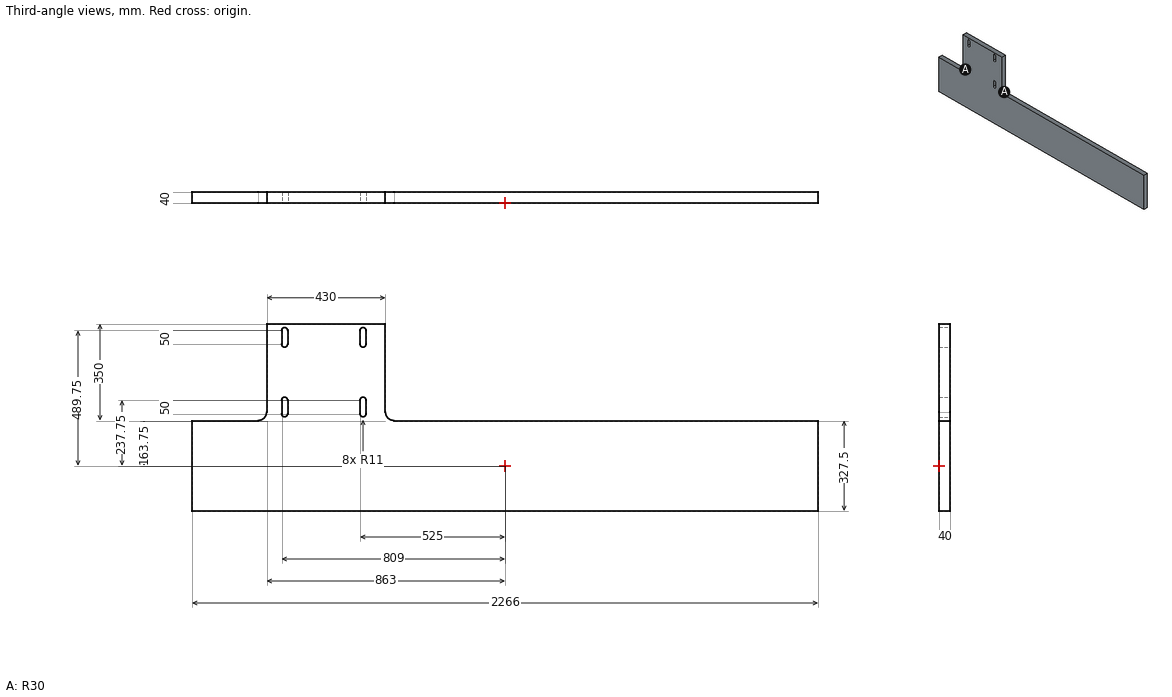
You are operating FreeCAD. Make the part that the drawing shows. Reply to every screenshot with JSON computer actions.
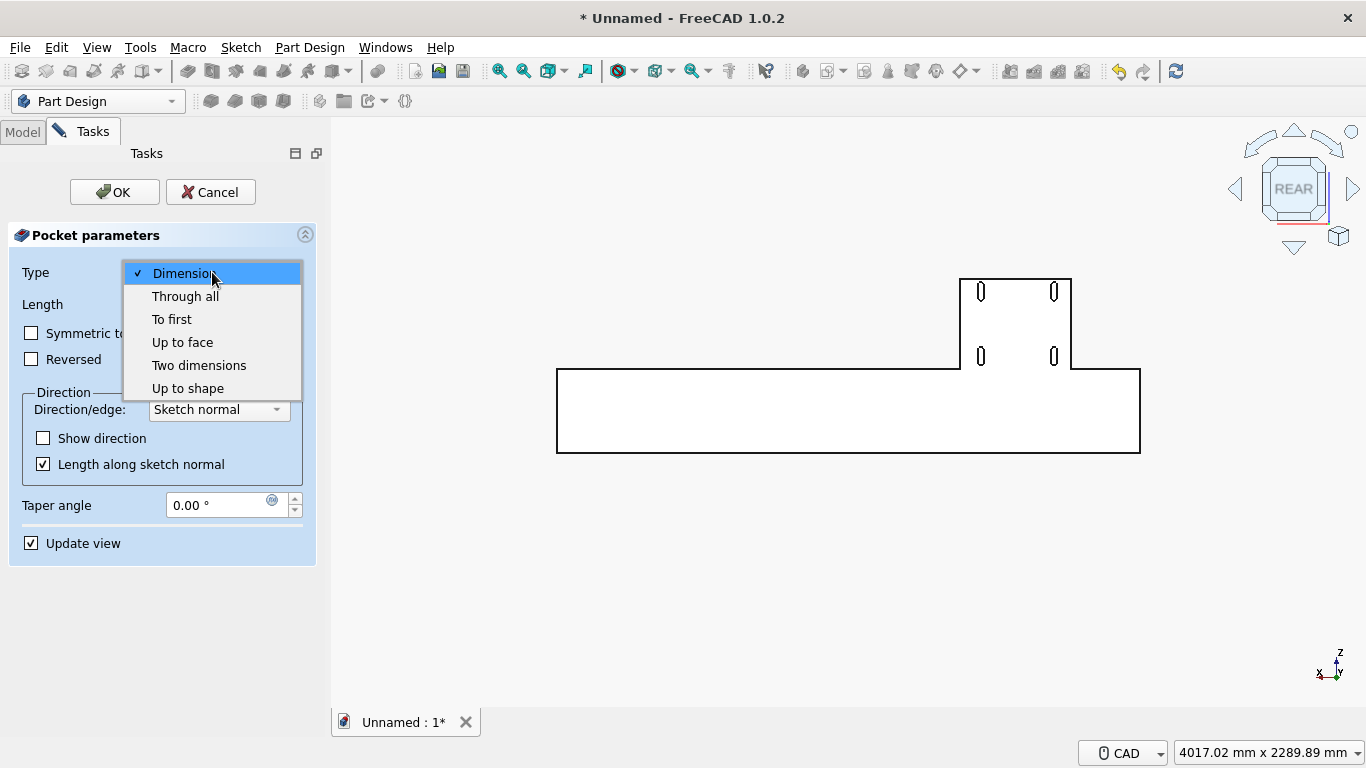
{"action": "left_click", "coordinate": [212, 296]}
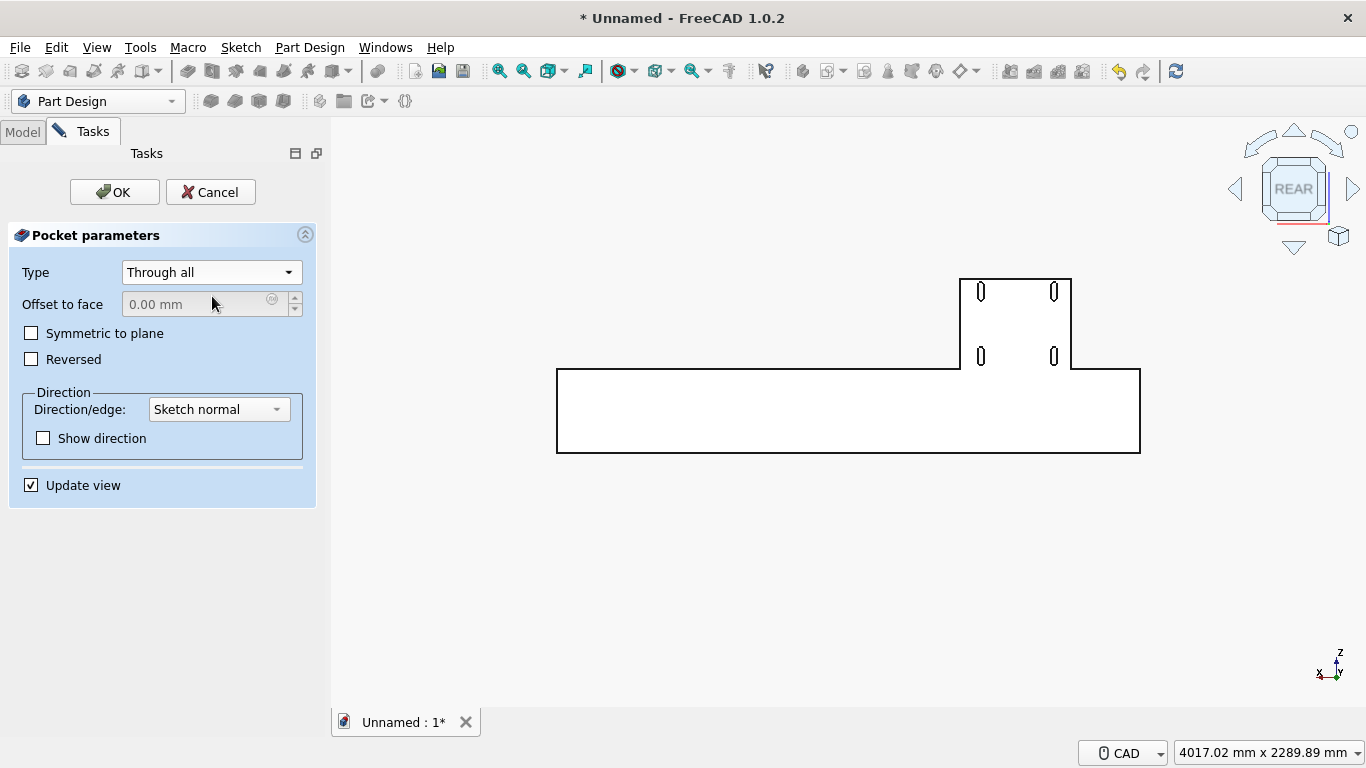
{"action": "left_click", "coordinate": [115, 192]}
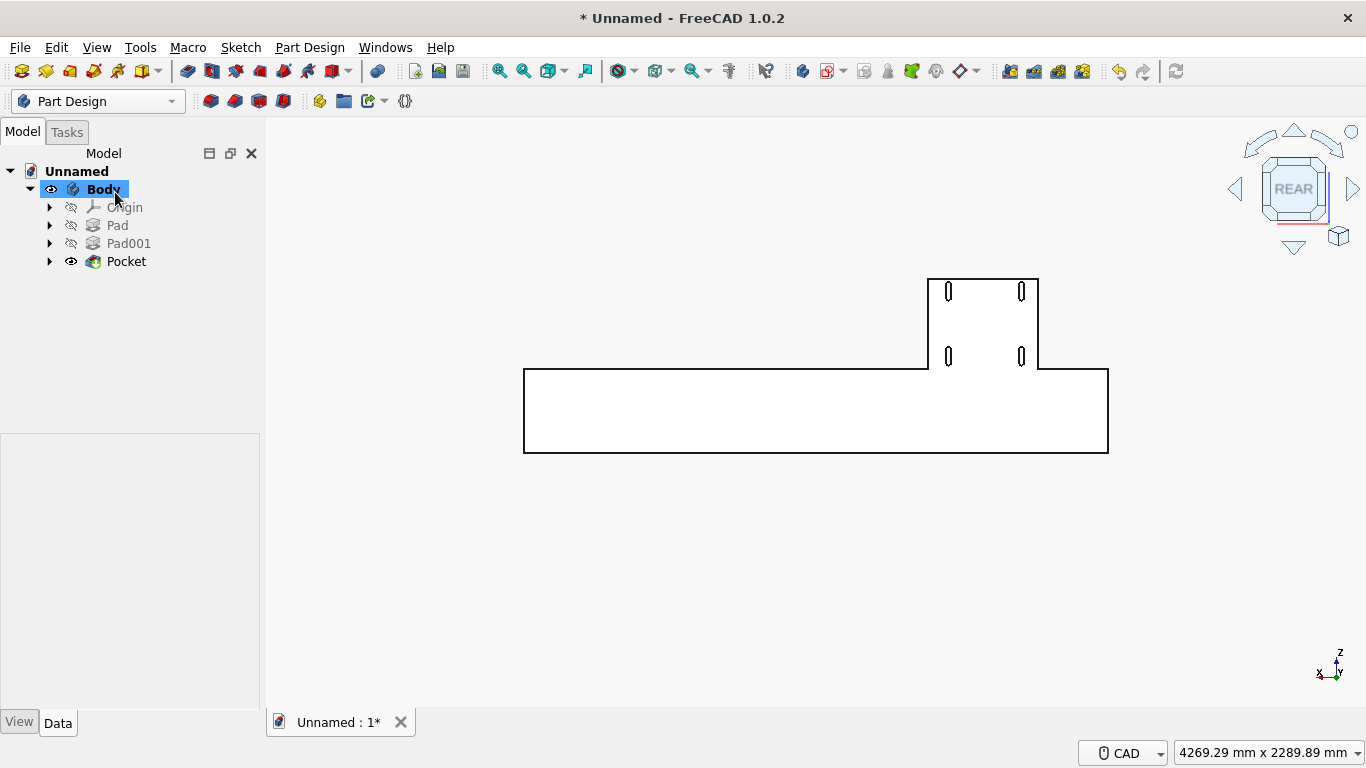
{"action": "scroll", "coordinate": [928, 368], "scroll_direction": "up", "scroll_amount": 7}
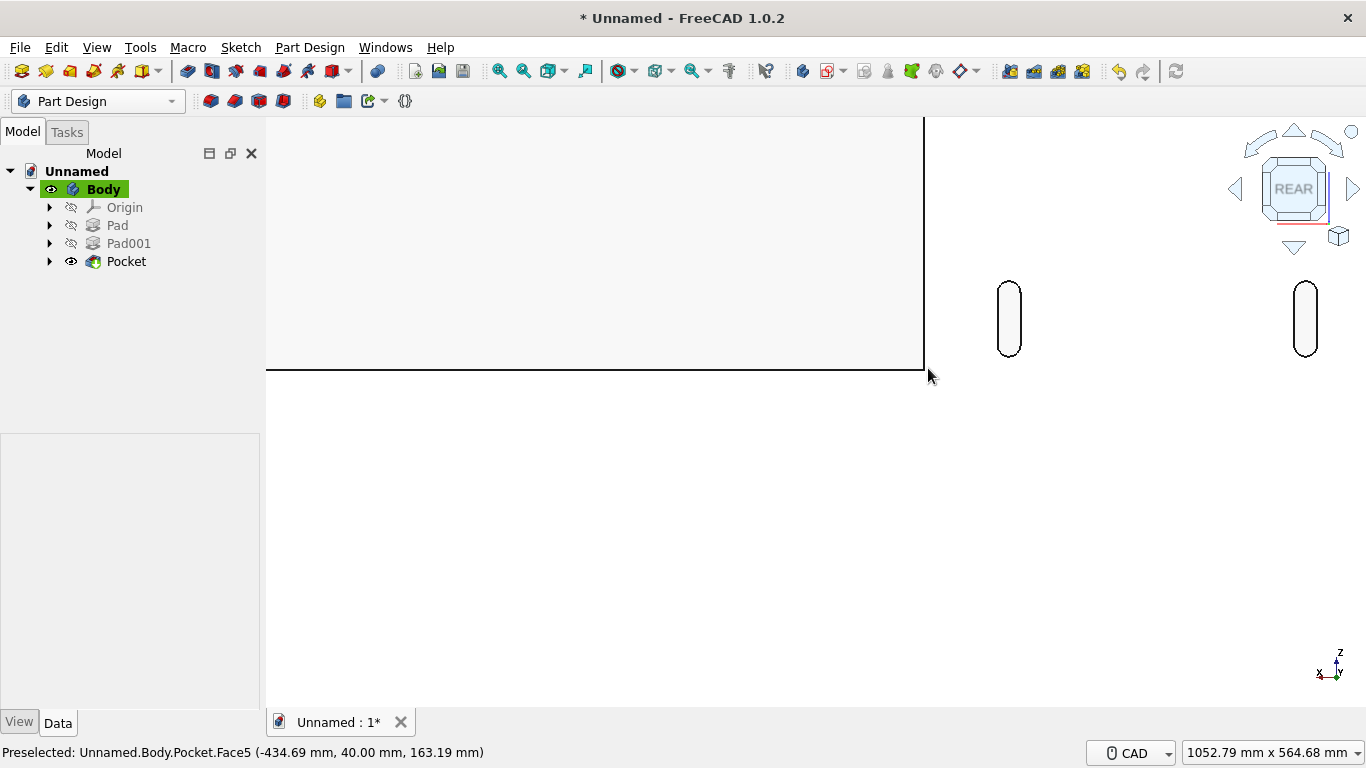
{"action": "left_click", "coordinate": [500, 72]}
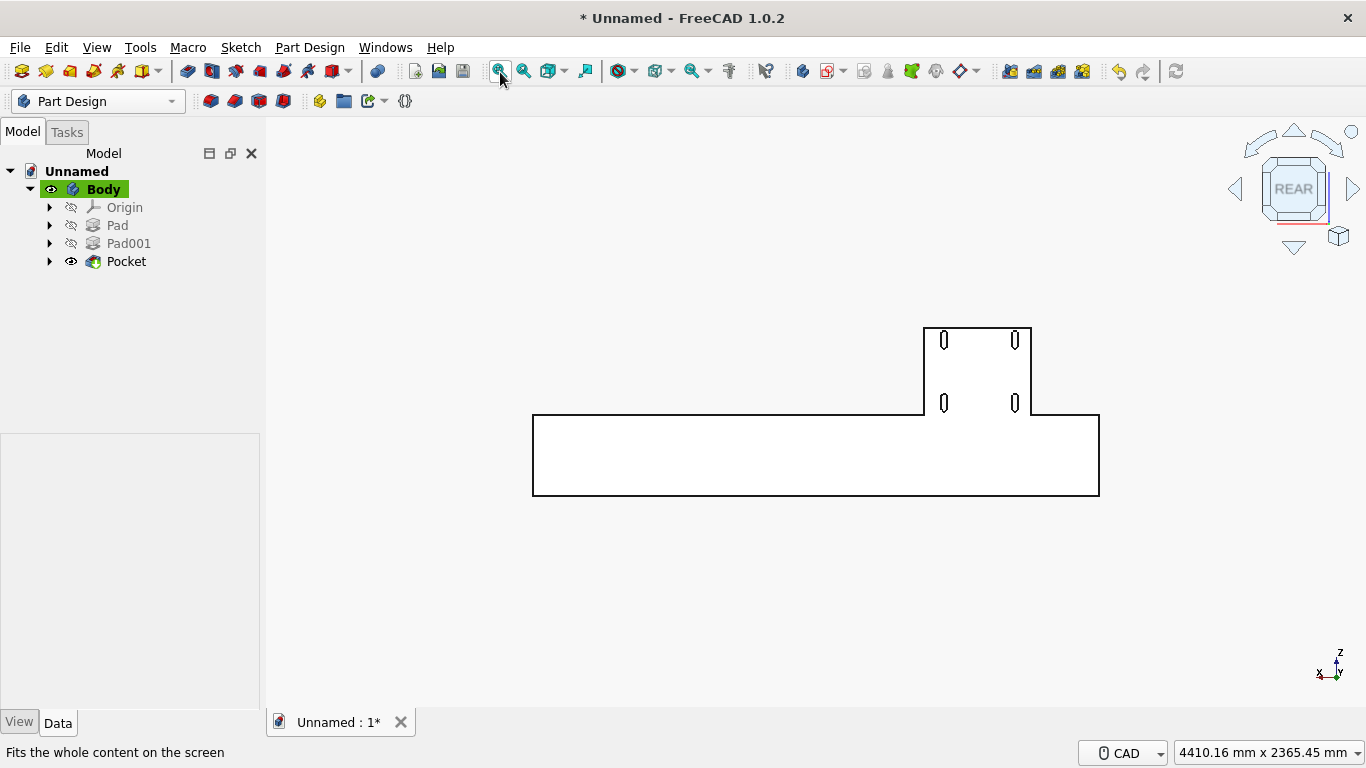
{"action": "key", "text": "0"}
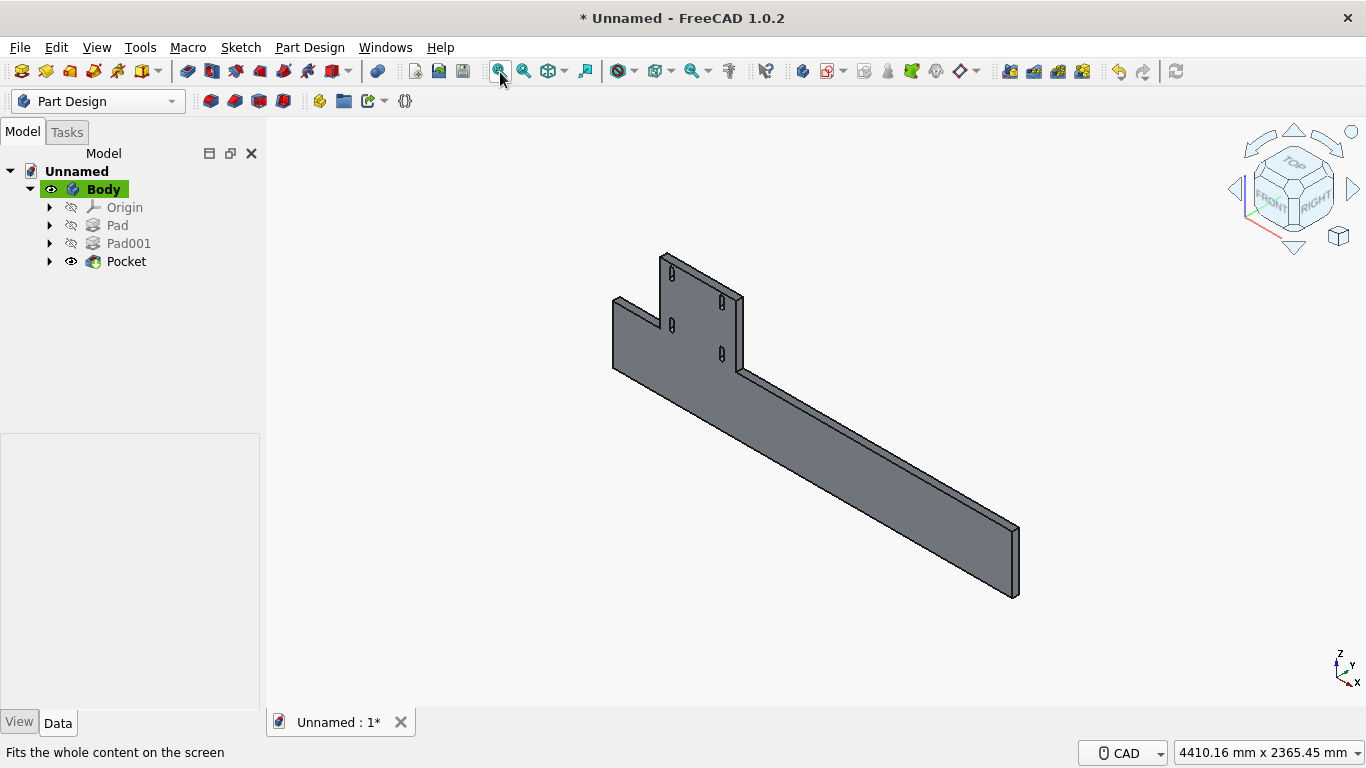
{"action": "scroll", "coordinate": [740, 369], "scroll_direction": "up", "scroll_amount": 7}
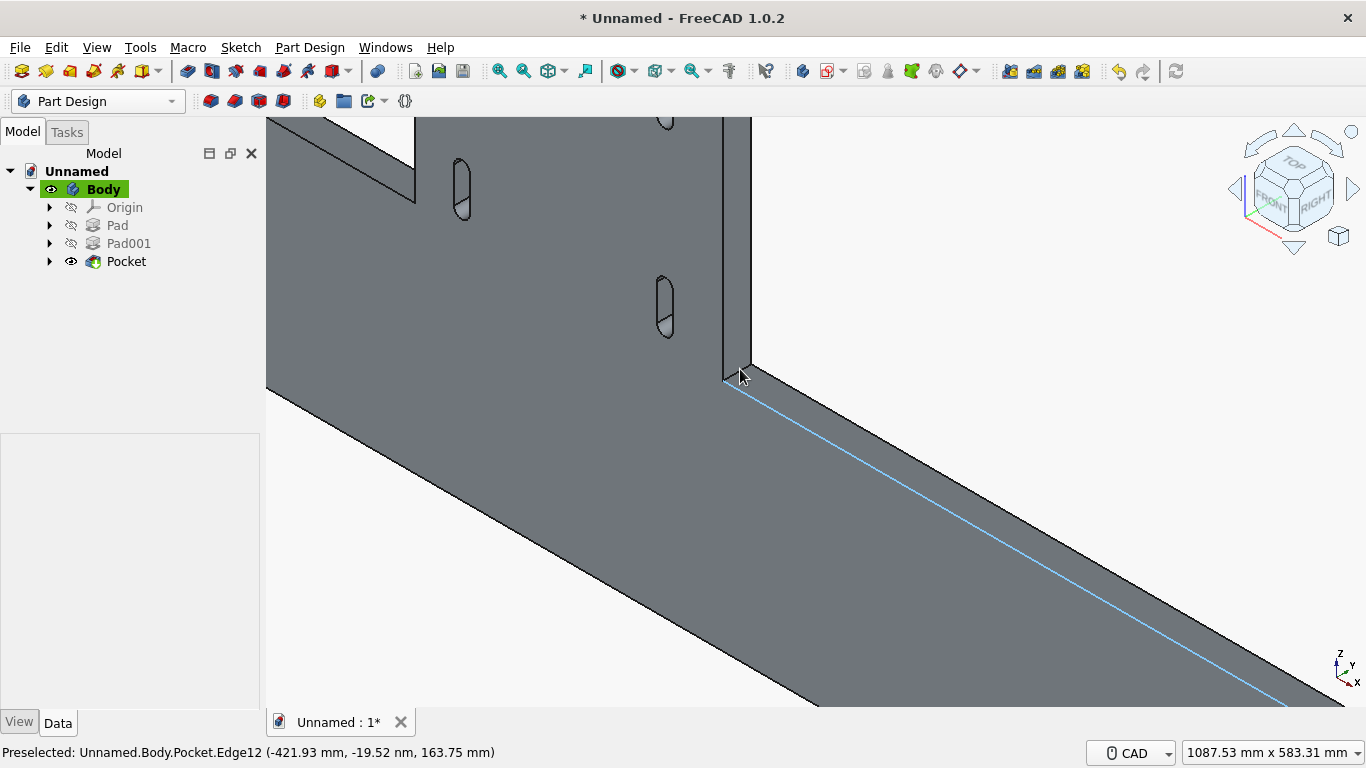
{"action": "left_click", "coordinate": [500, 72]}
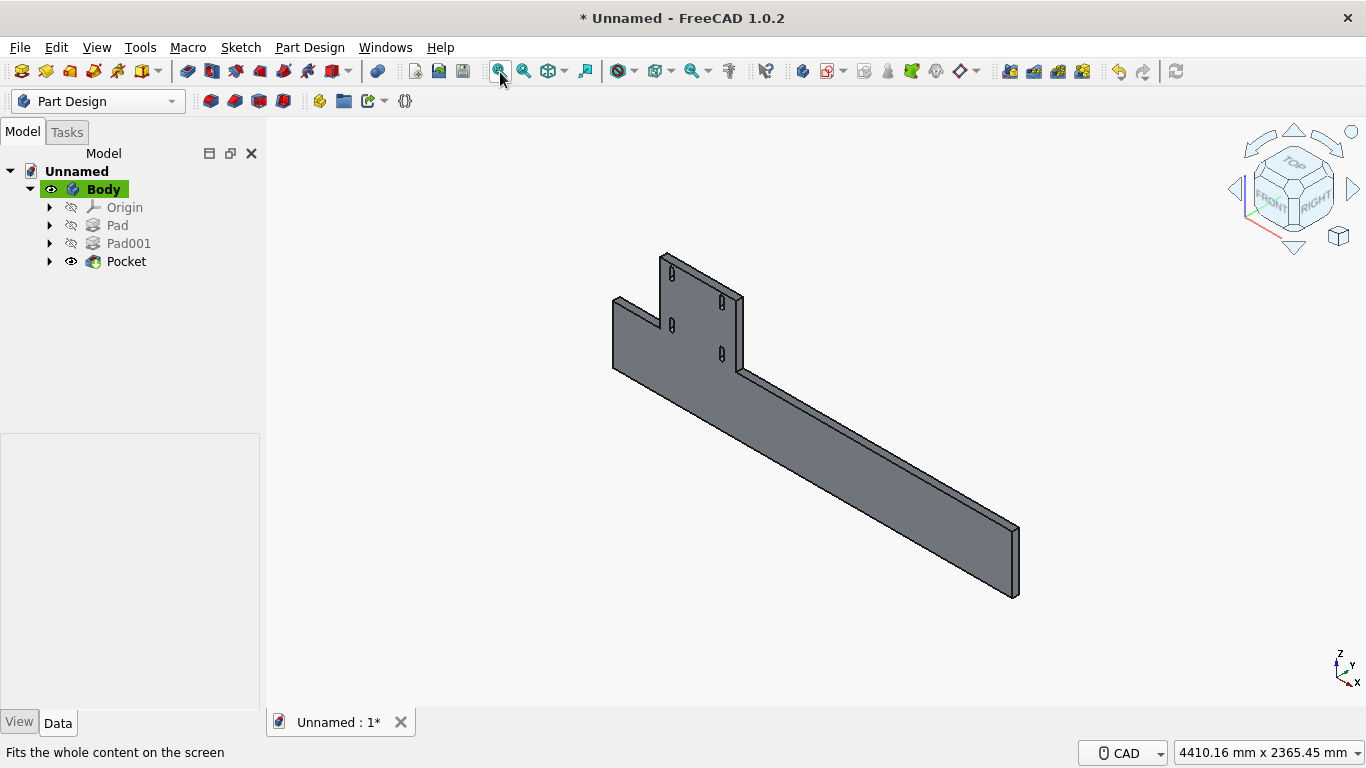
{"action": "key", "text": "2"}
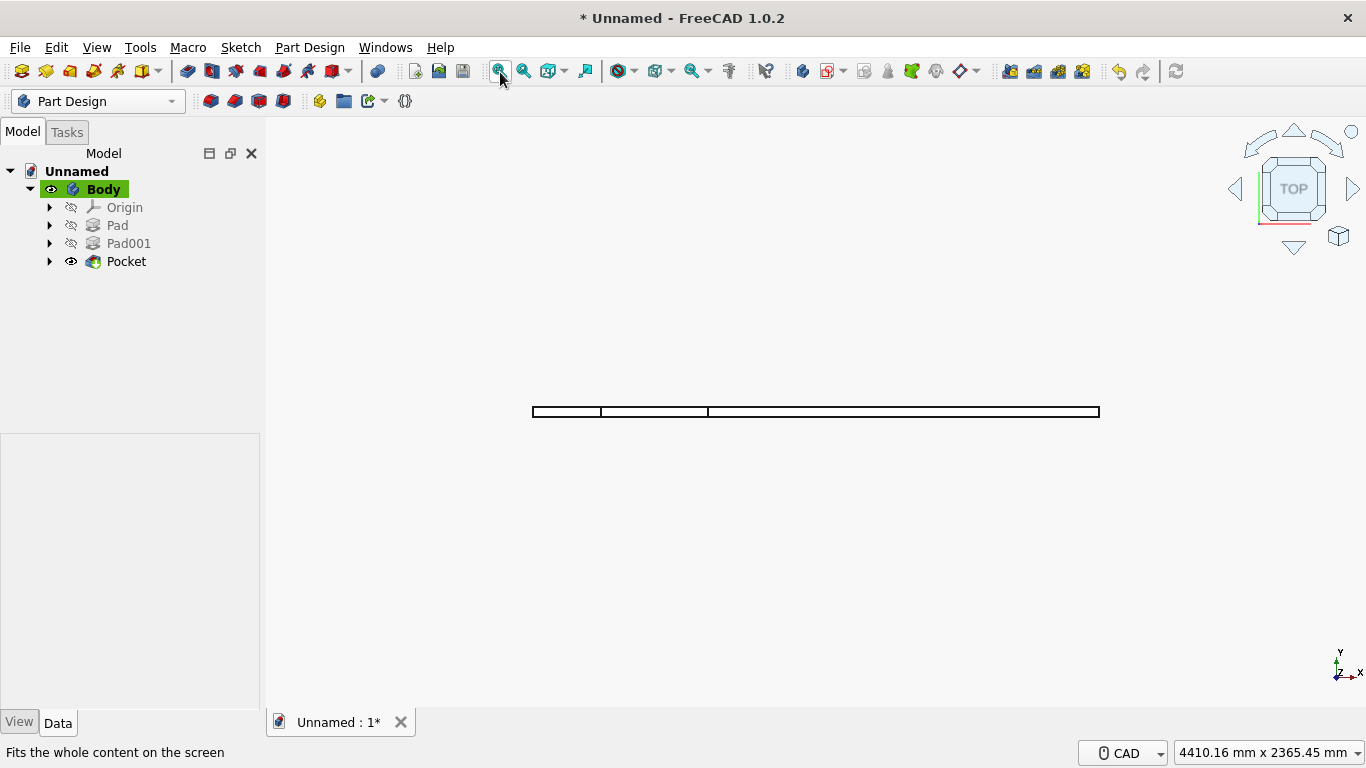
{"action": "scroll", "coordinate": [708, 411], "scroll_direction": "up", "scroll_amount": 7}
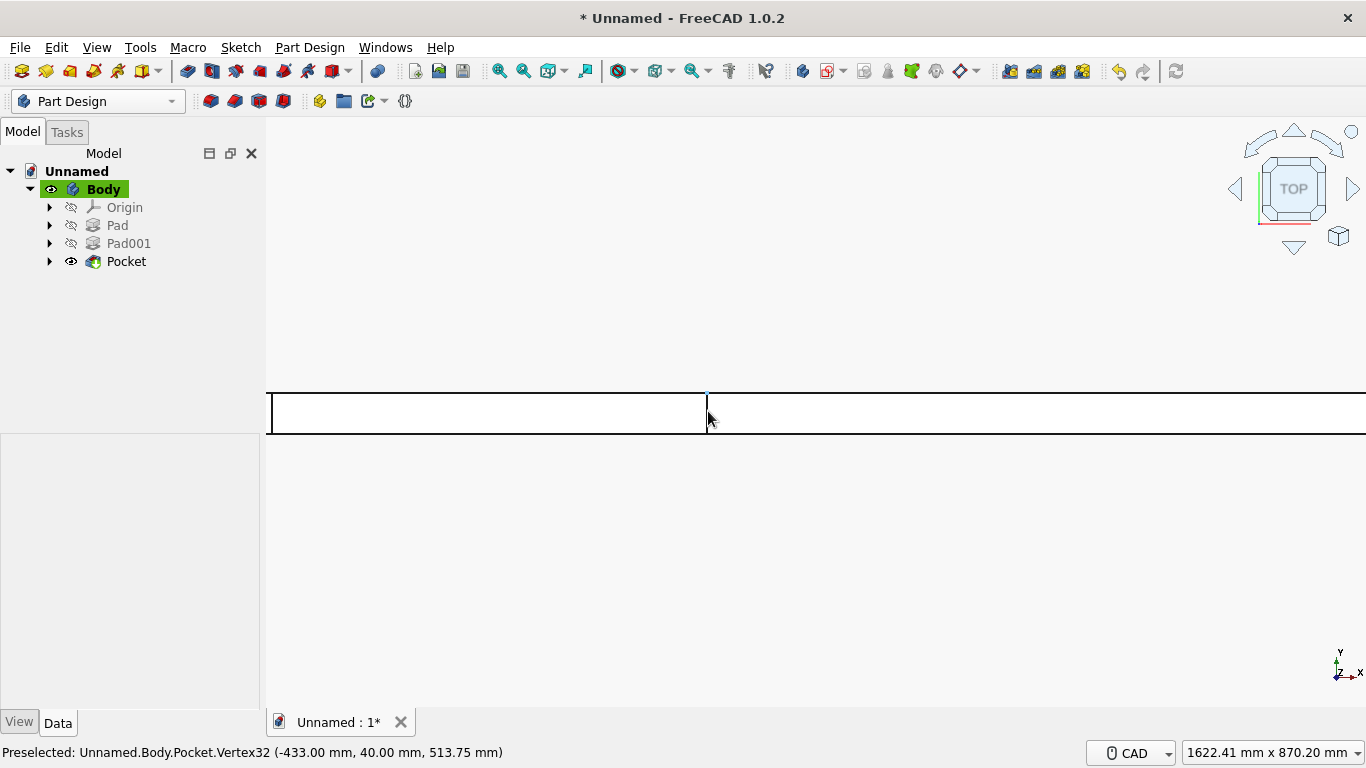
{"action": "key", "text": "v f"}